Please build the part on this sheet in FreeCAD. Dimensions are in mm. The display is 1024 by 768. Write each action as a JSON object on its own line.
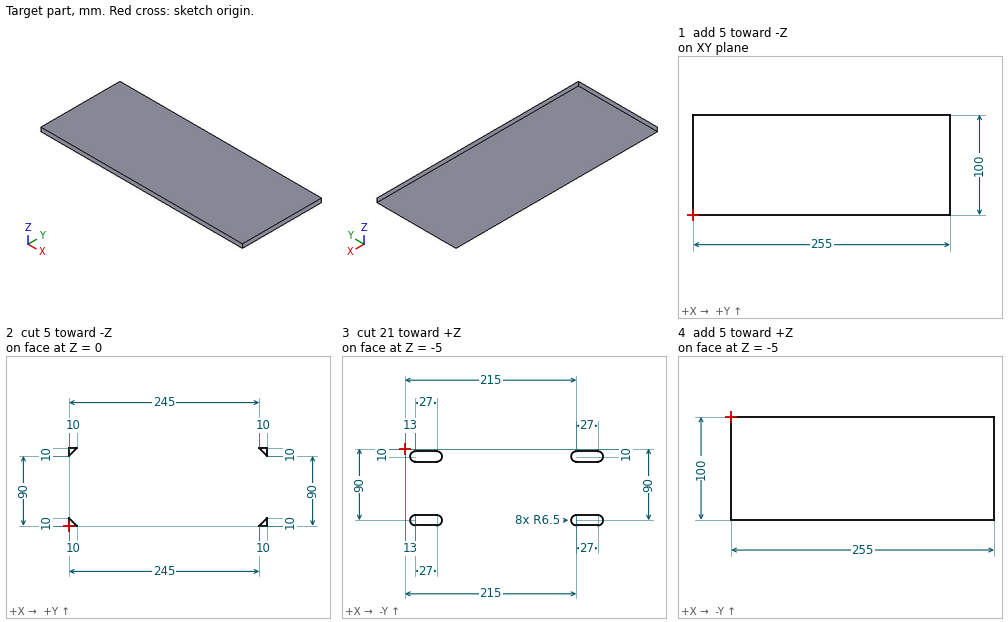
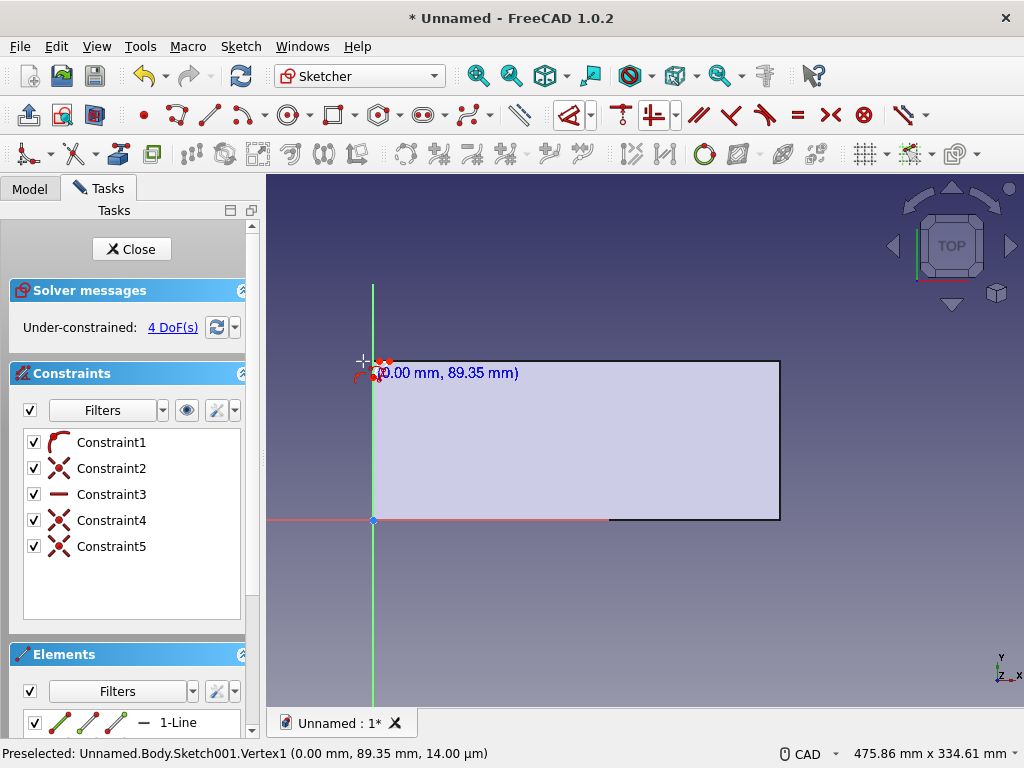
{"action": "left_click", "coordinate": [764, 361]}
{"action": "left_click", "coordinate": [780, 377]}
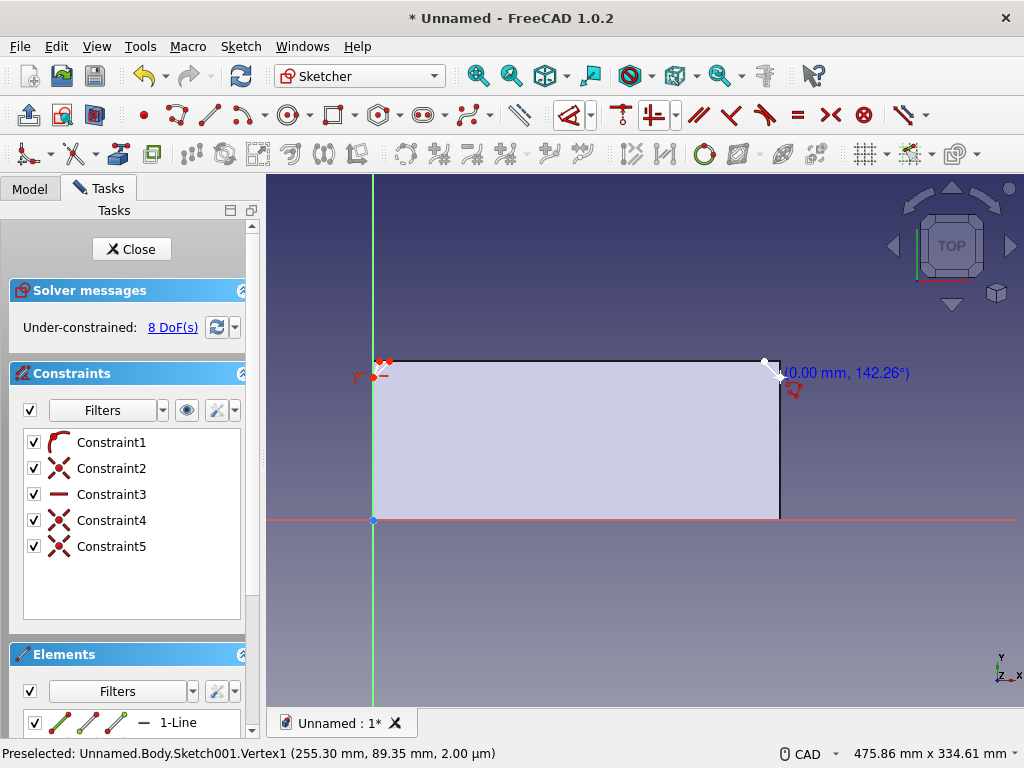
{"action": "scroll", "coordinate": [780, 361], "scroll_direction": "up", "scroll_amount": 2}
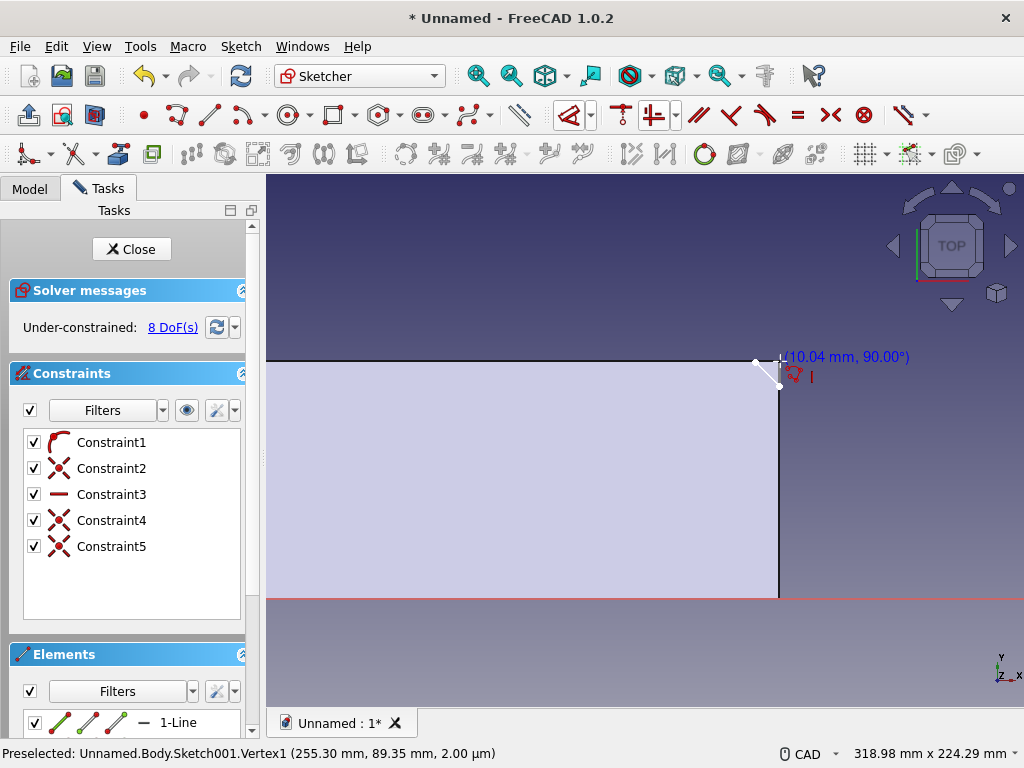
{"action": "left_click", "coordinate": [780, 361]}
{"action": "left_click", "coordinate": [756, 362]}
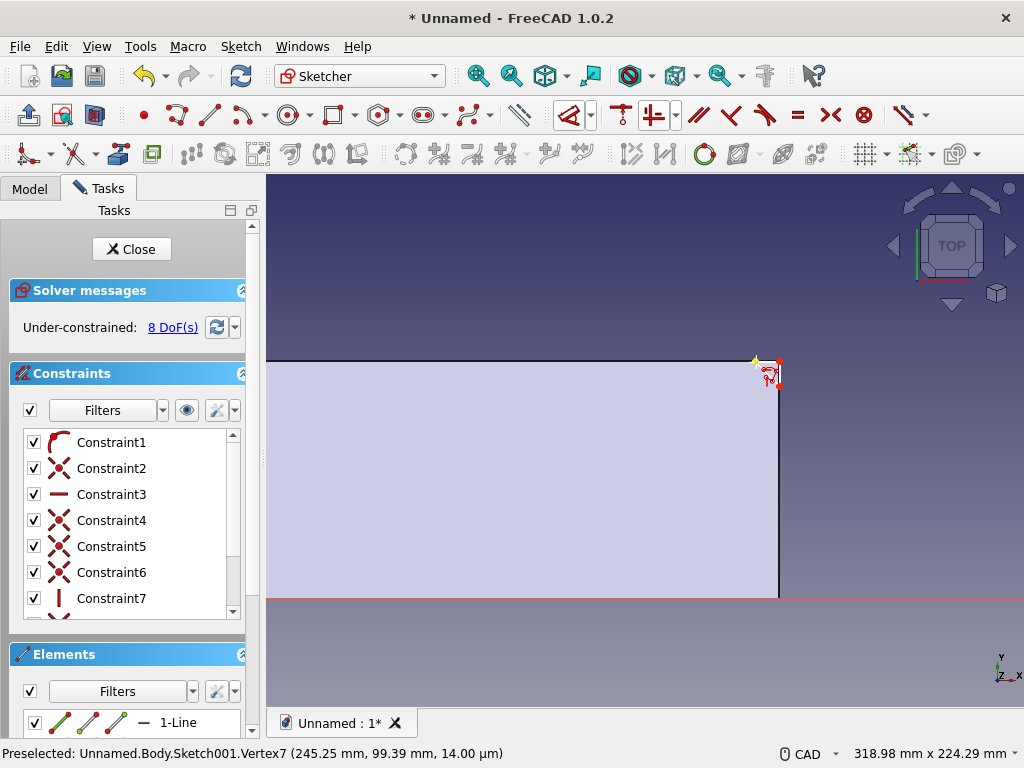
{"action": "left_click", "coordinate": [755, 599]}
{"action": "left_click", "coordinate": [779, 590]}
{"action": "left_click", "coordinate": [779, 575]}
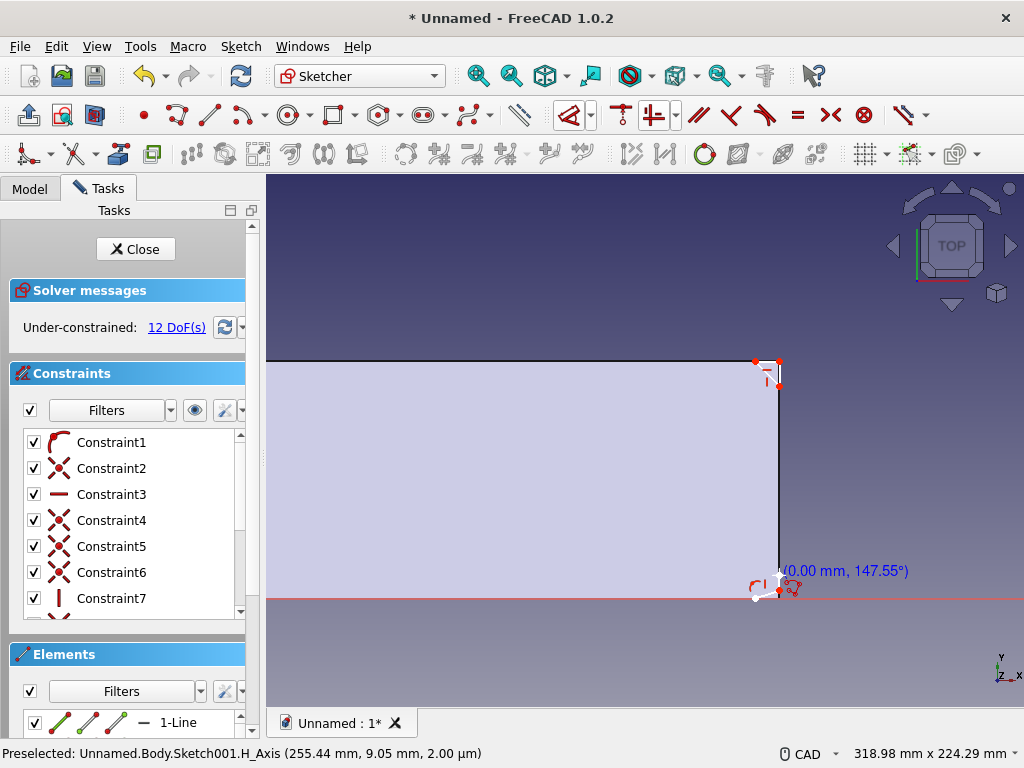
{"action": "scroll", "coordinate": [755, 599], "scroll_direction": "up", "scroll_amount": 2}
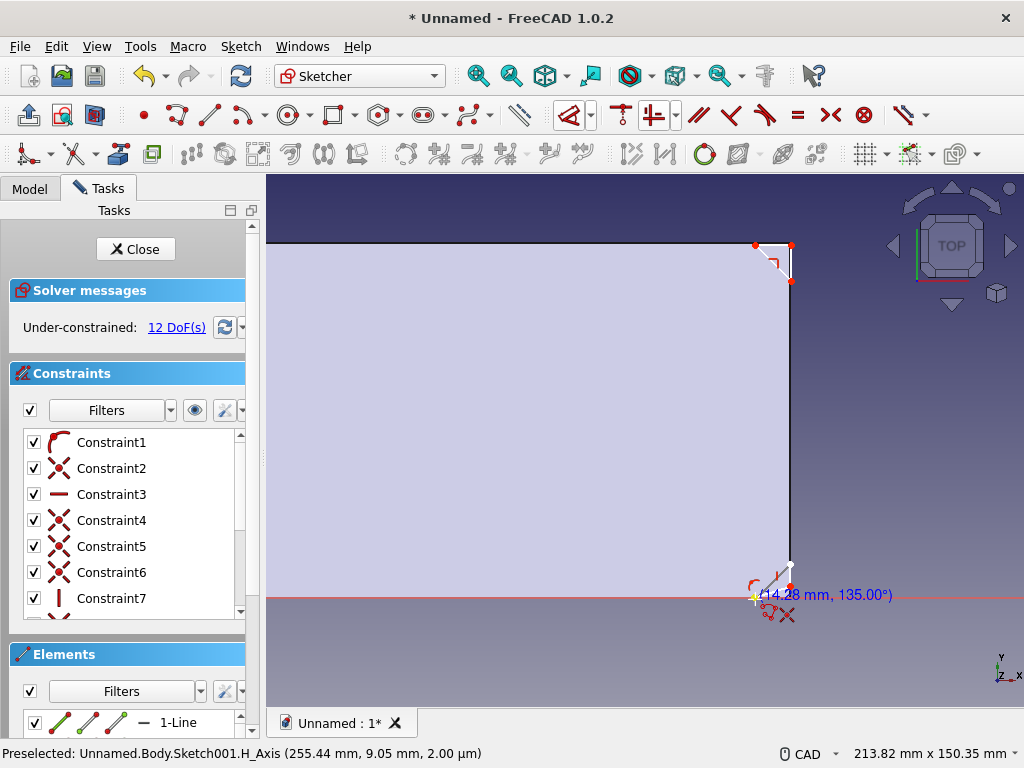
{"action": "left_click", "coordinate": [755, 598]}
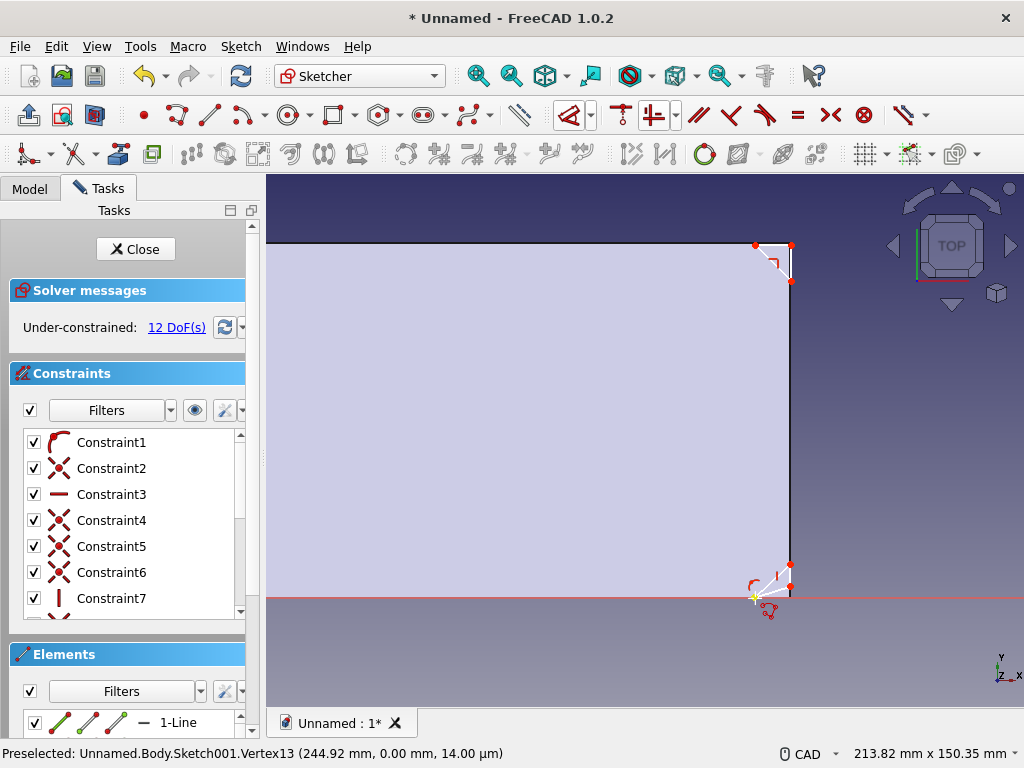
{"action": "scroll", "coordinate": [771, 457], "scroll_direction": "down", "scroll_amount": 4}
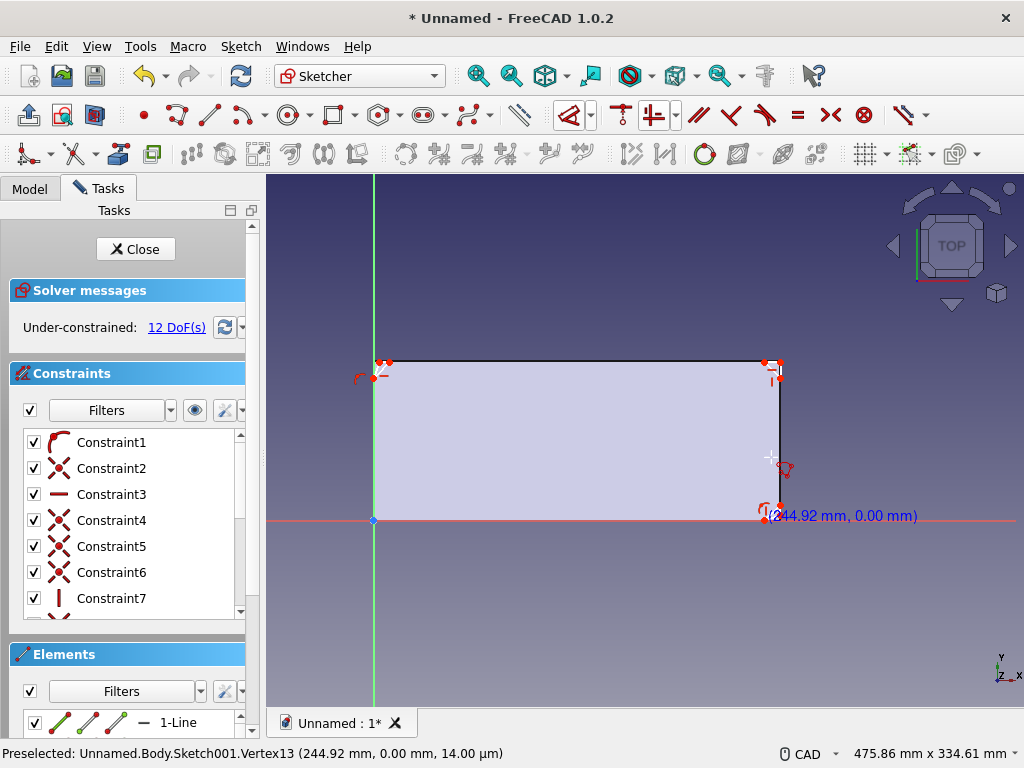
{"action": "left_click", "coordinate": [374, 521]}
{"action": "left_click", "coordinate": [390, 512]}
{"action": "left_click", "coordinate": [383, 505]}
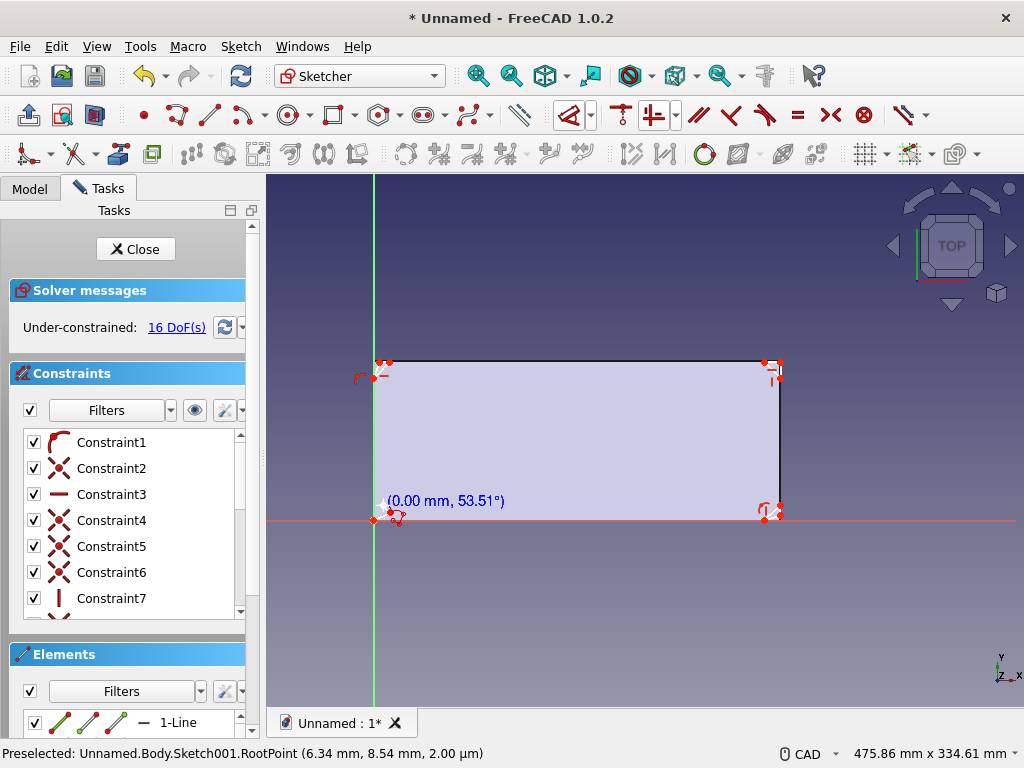
{"action": "scroll", "coordinate": [374, 521], "scroll_direction": "up", "scroll_amount": 4}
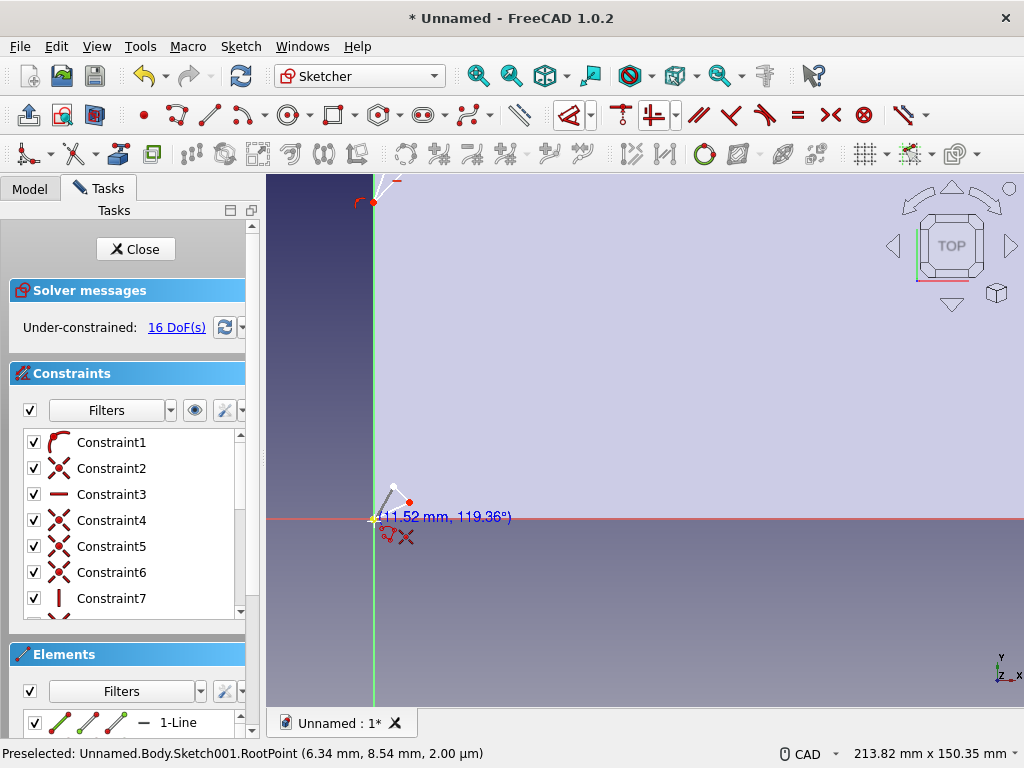
{"action": "left_click", "coordinate": [374, 519]}
{"action": "key", "text": "Escape"}
{"action": "key", "text": "Escape"}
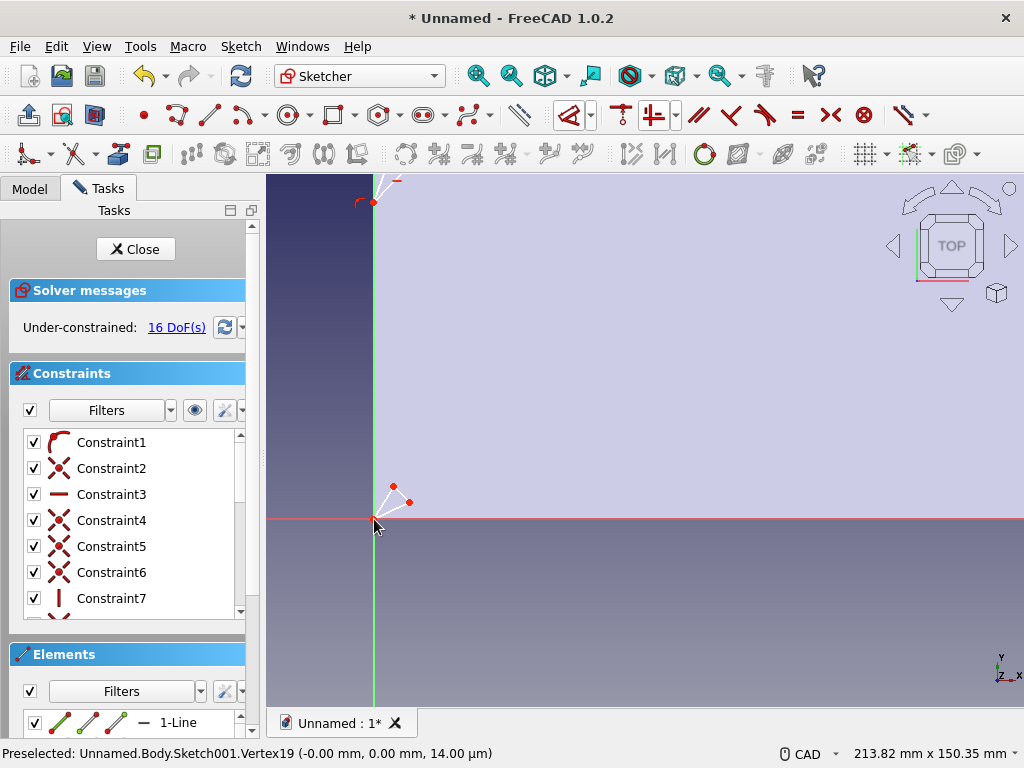
{"action": "scroll", "coordinate": [373, 521], "scroll_direction": "down", "scroll_amount": 4}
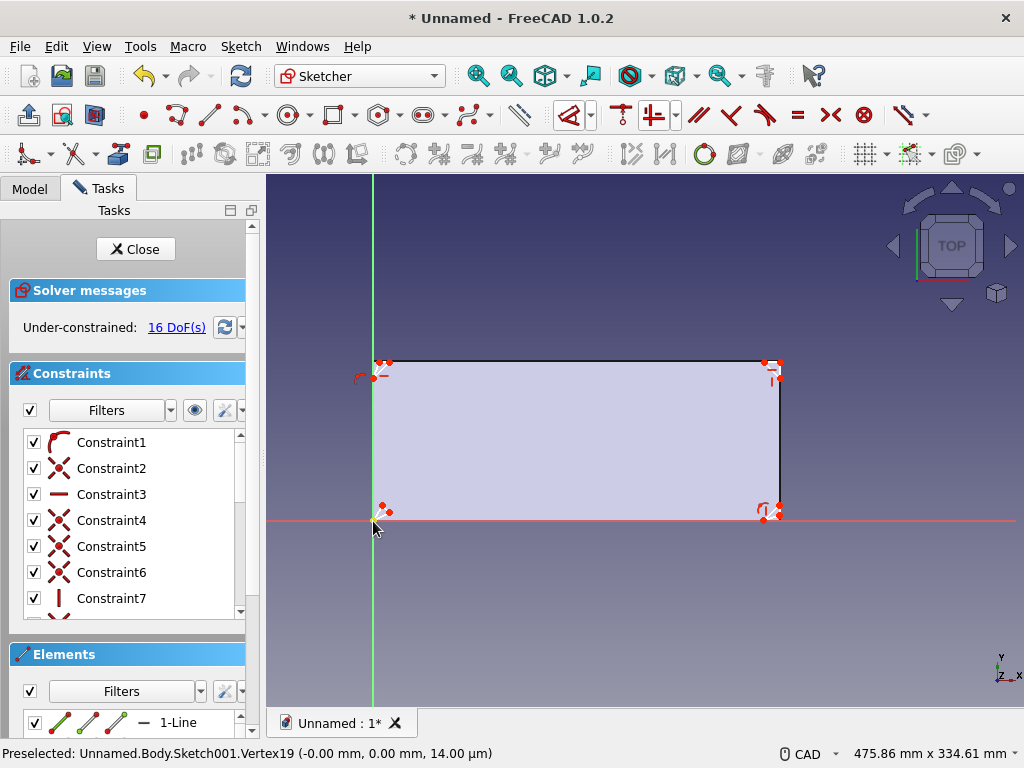
{"action": "scroll", "coordinate": [377, 367], "scroll_direction": "up", "scroll_amount": 7}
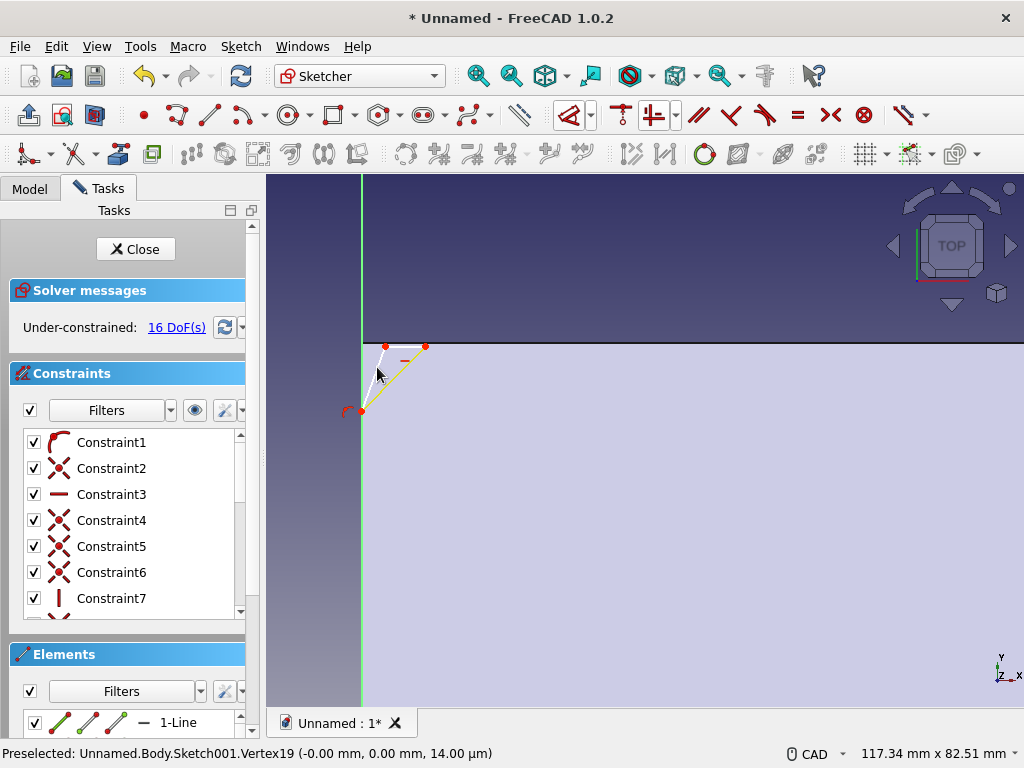
{"action": "left_click", "coordinate": [378, 366]}